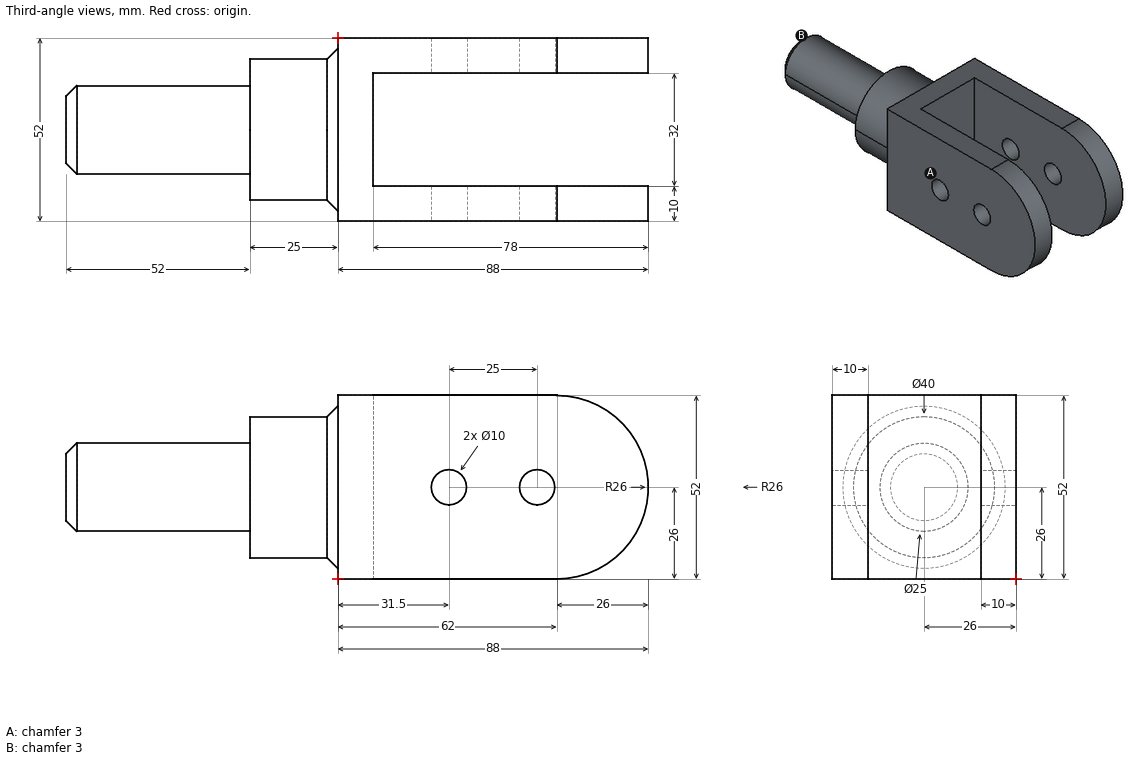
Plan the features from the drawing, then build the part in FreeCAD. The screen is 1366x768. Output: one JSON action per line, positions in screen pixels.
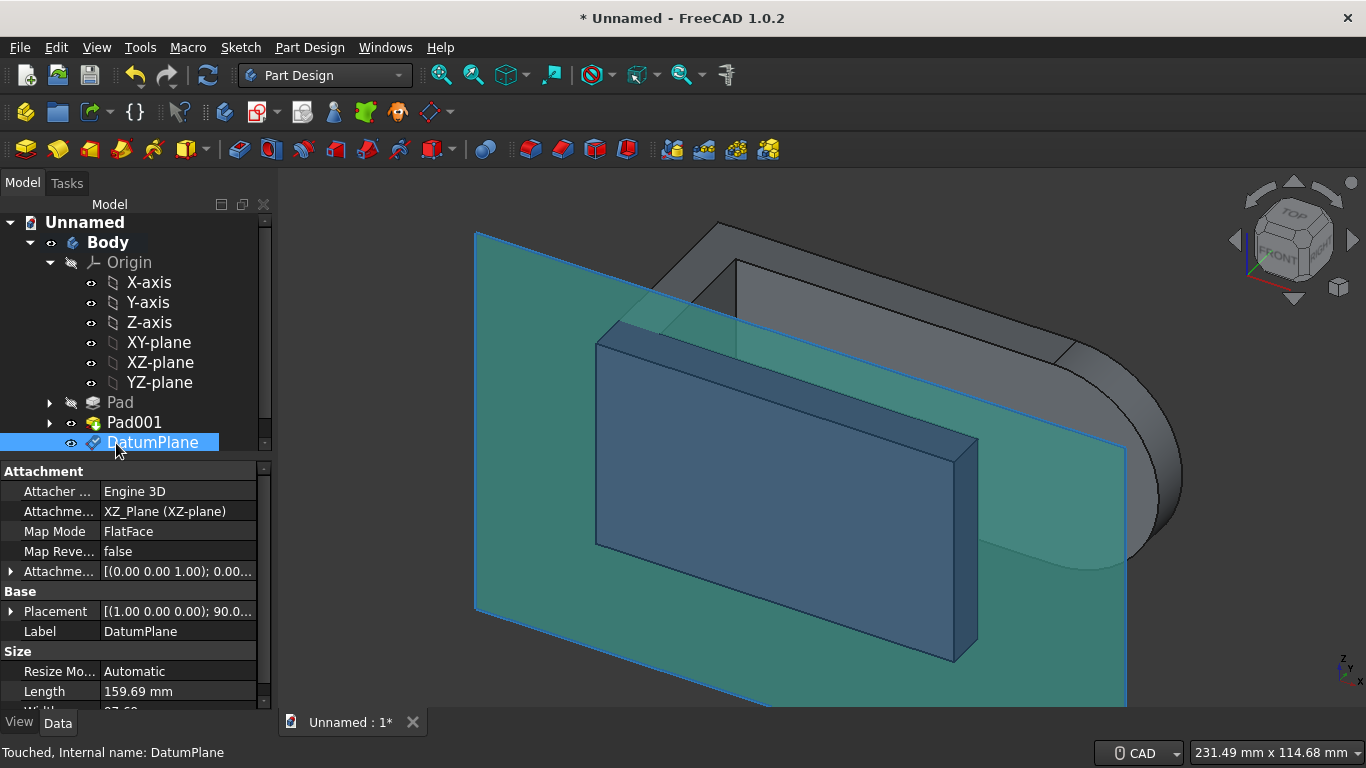
{"action": "left_click", "coordinate": [258, 112]}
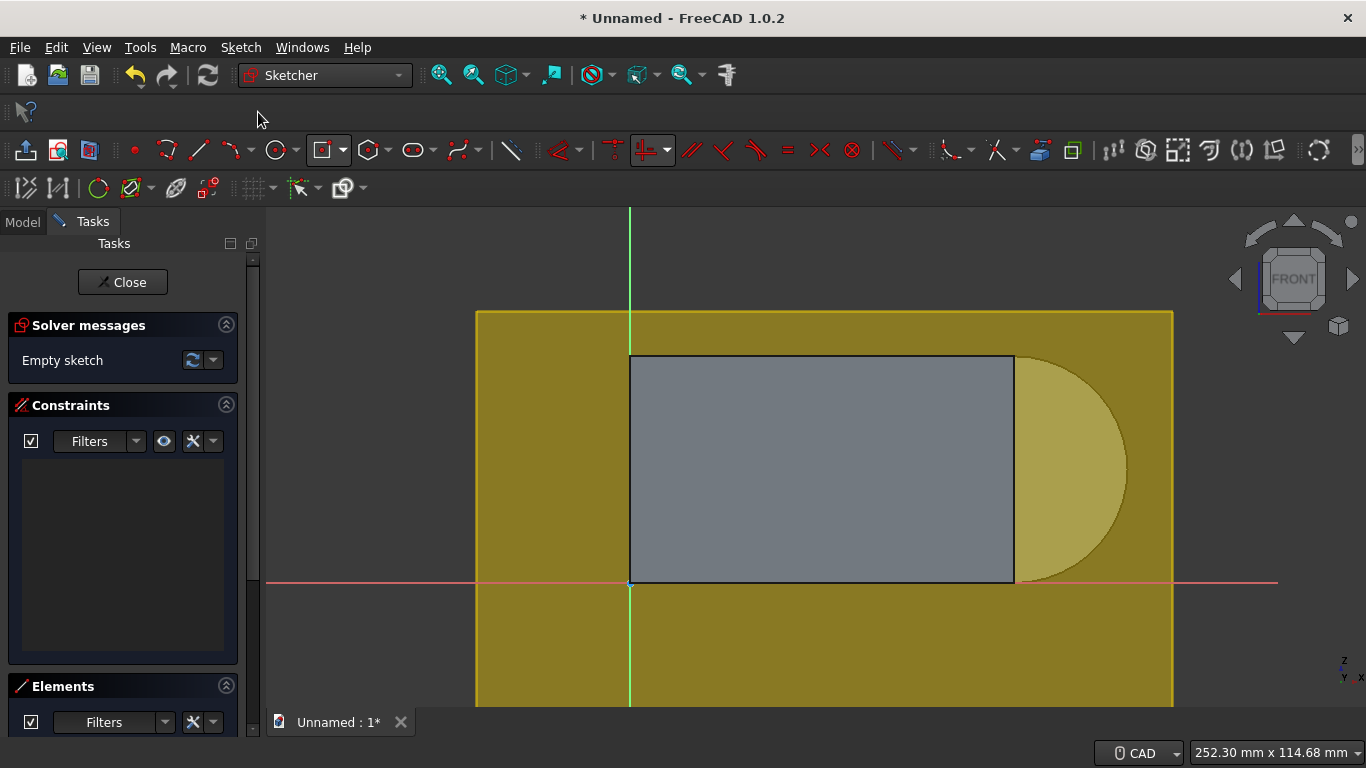
{"action": "left_click", "coordinate": [90, 150]}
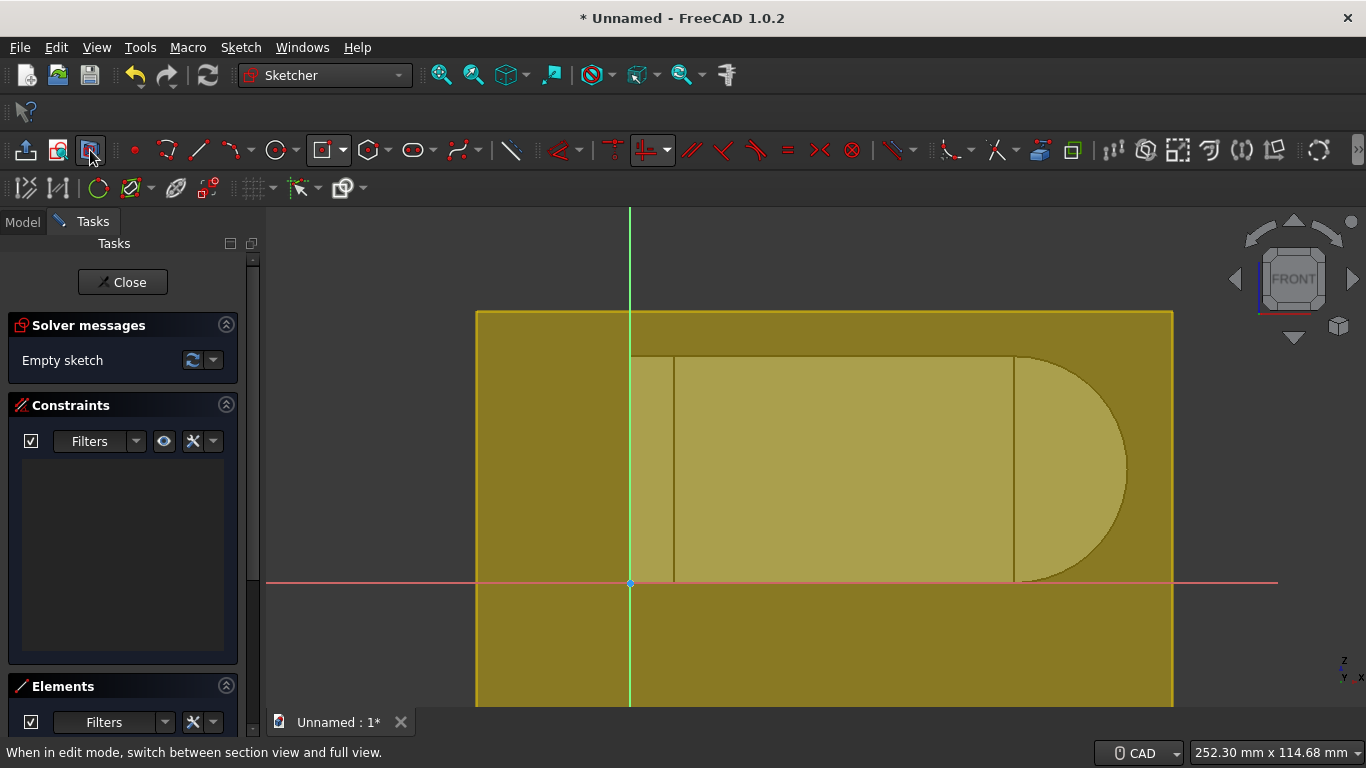
{"action": "left_click", "coordinate": [200, 150]}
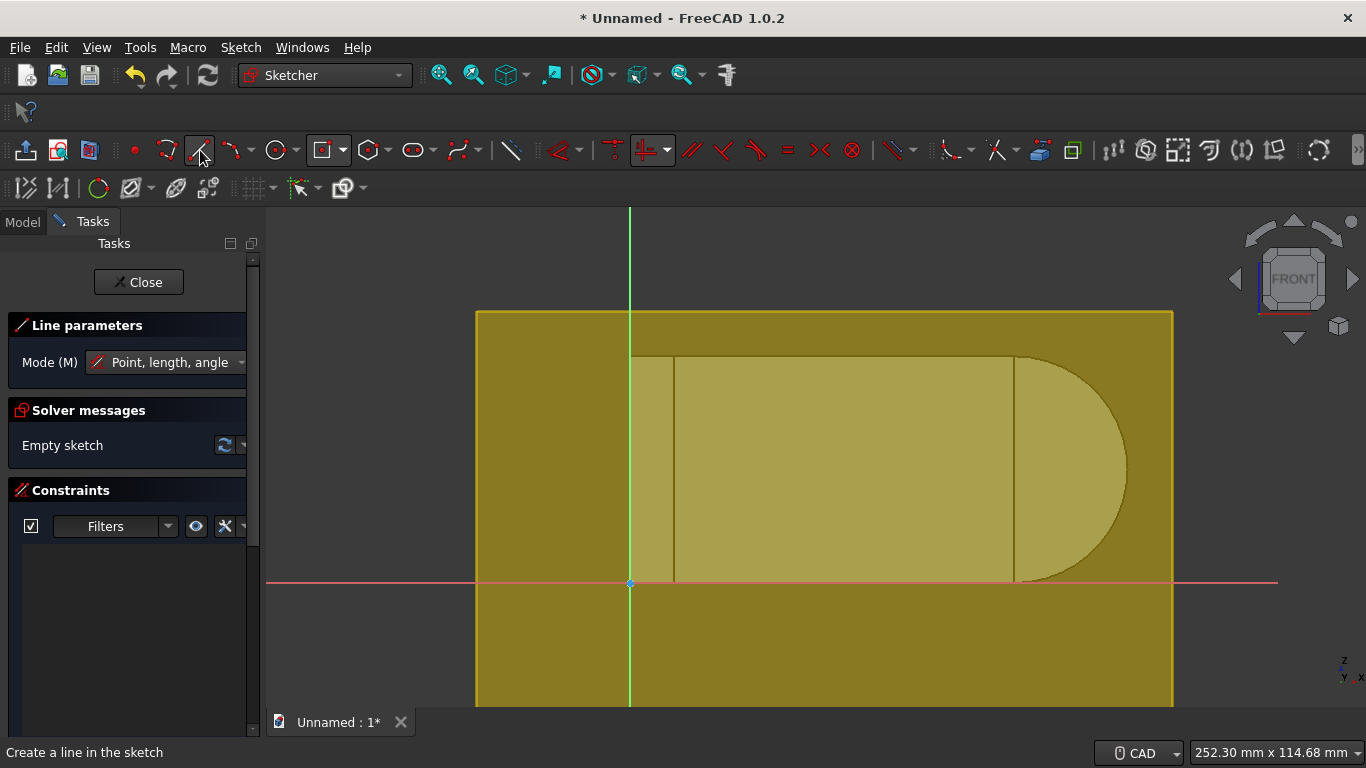
{"action": "left_click", "coordinate": [1014, 356]}
{"action": "left_click", "coordinate": [1014, 583]}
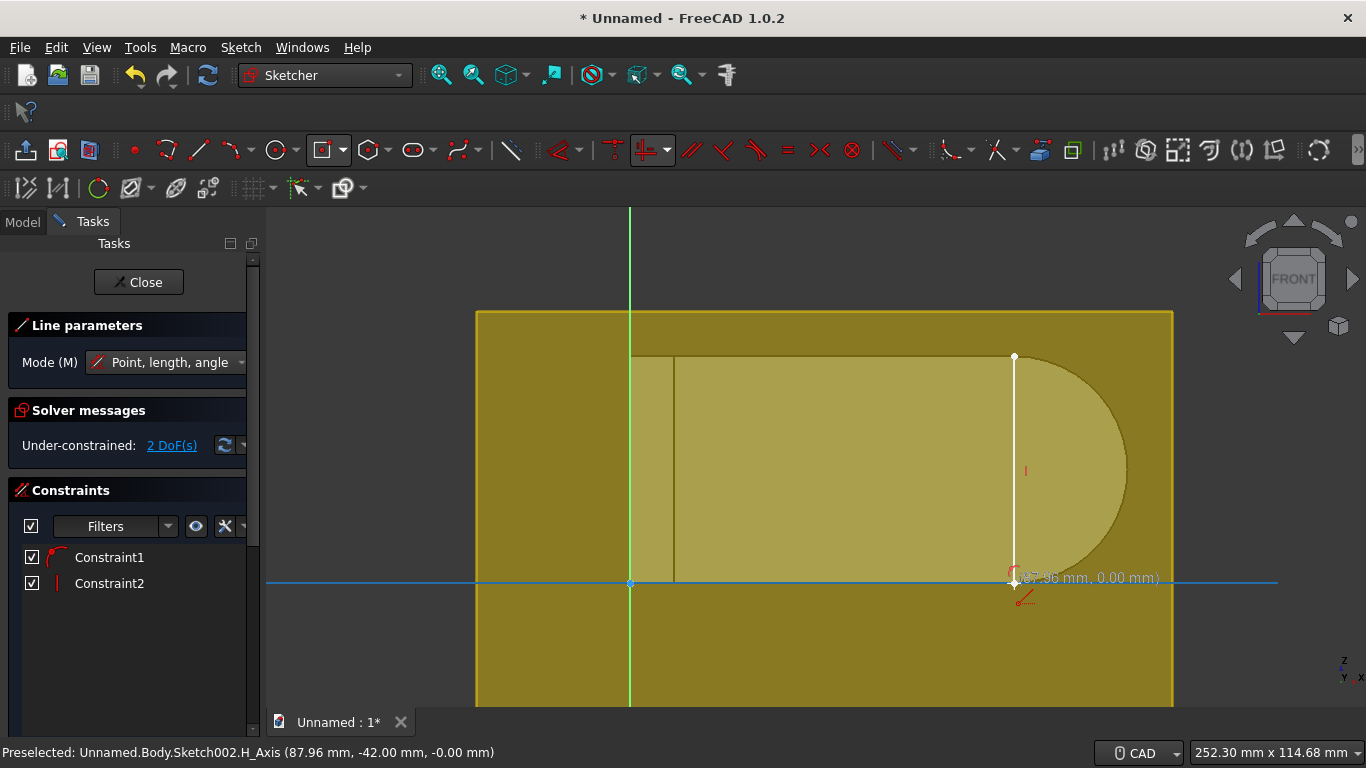
{"action": "left_click", "coordinate": [232, 150]}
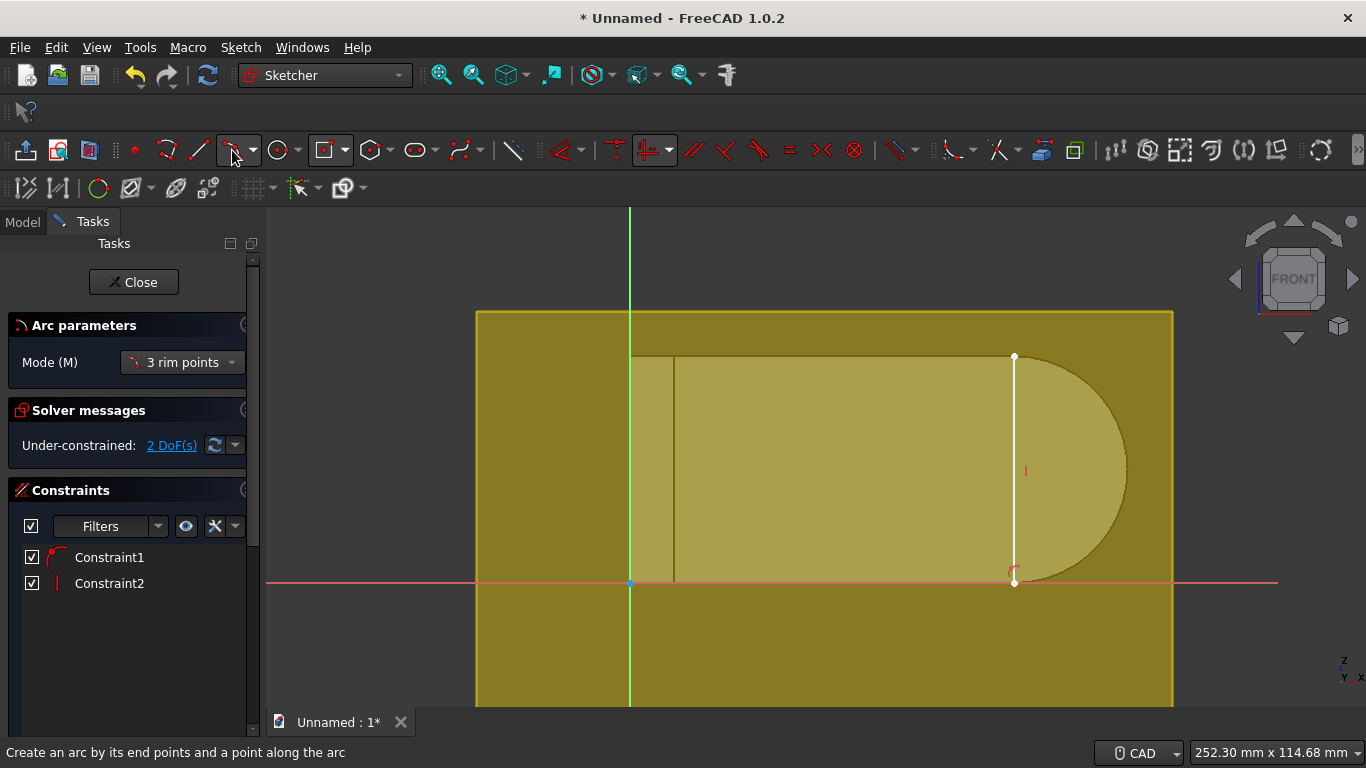
{"action": "left_click", "coordinate": [1014, 583]}
{"action": "left_click", "coordinate": [1014, 357]}
{"action": "left_click", "coordinate": [1128, 470]}
{"action": "key", "text": "Escape"}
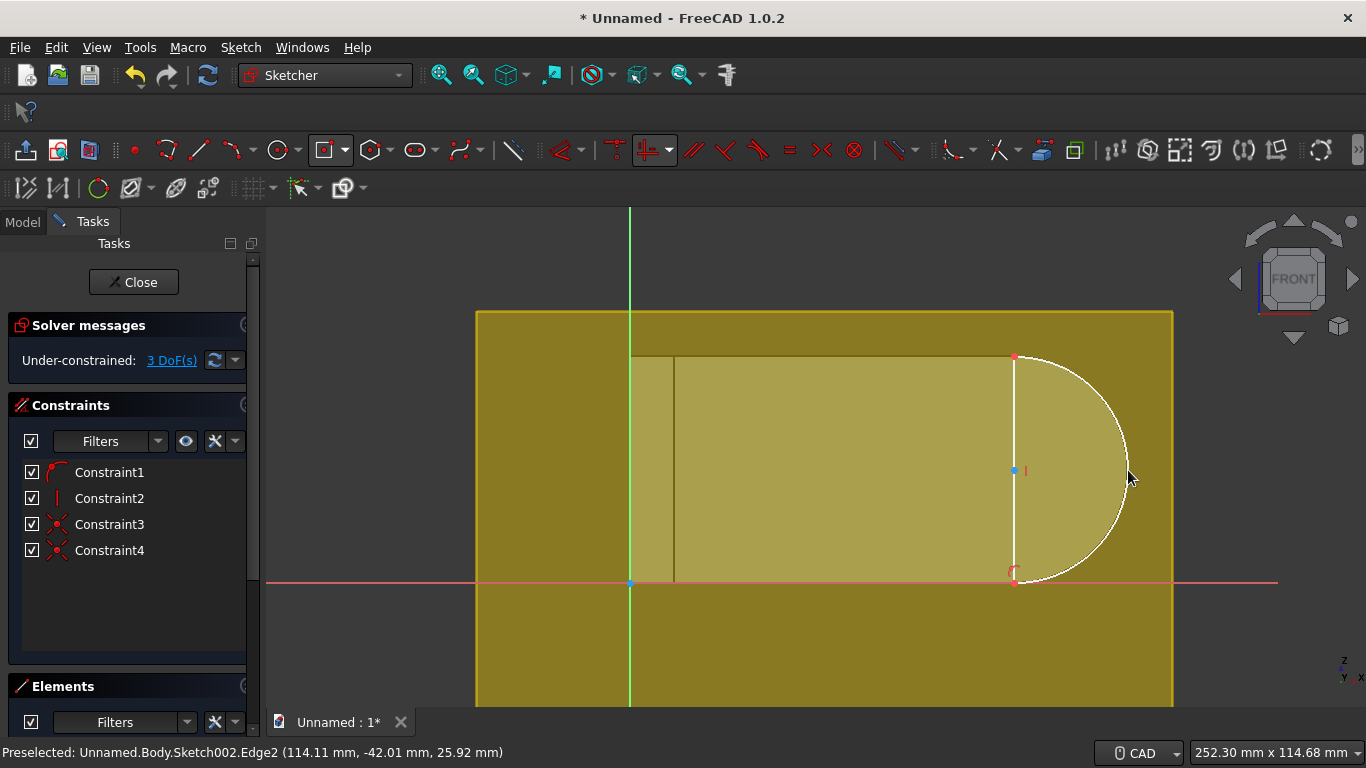
{"action": "left_click", "coordinate": [560, 150]}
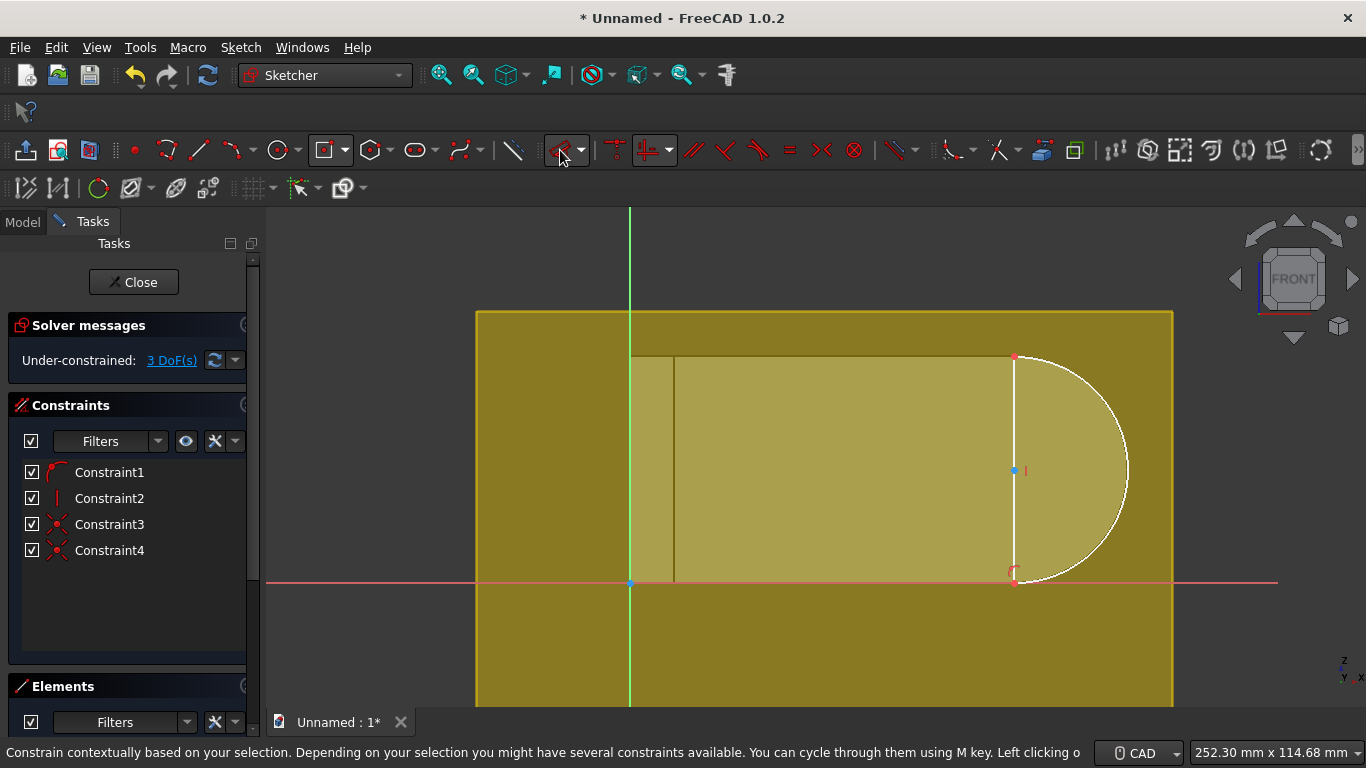
{"action": "left_click", "coordinate": [1106, 537]}
{"action": "left_click", "coordinate": [1132, 556]}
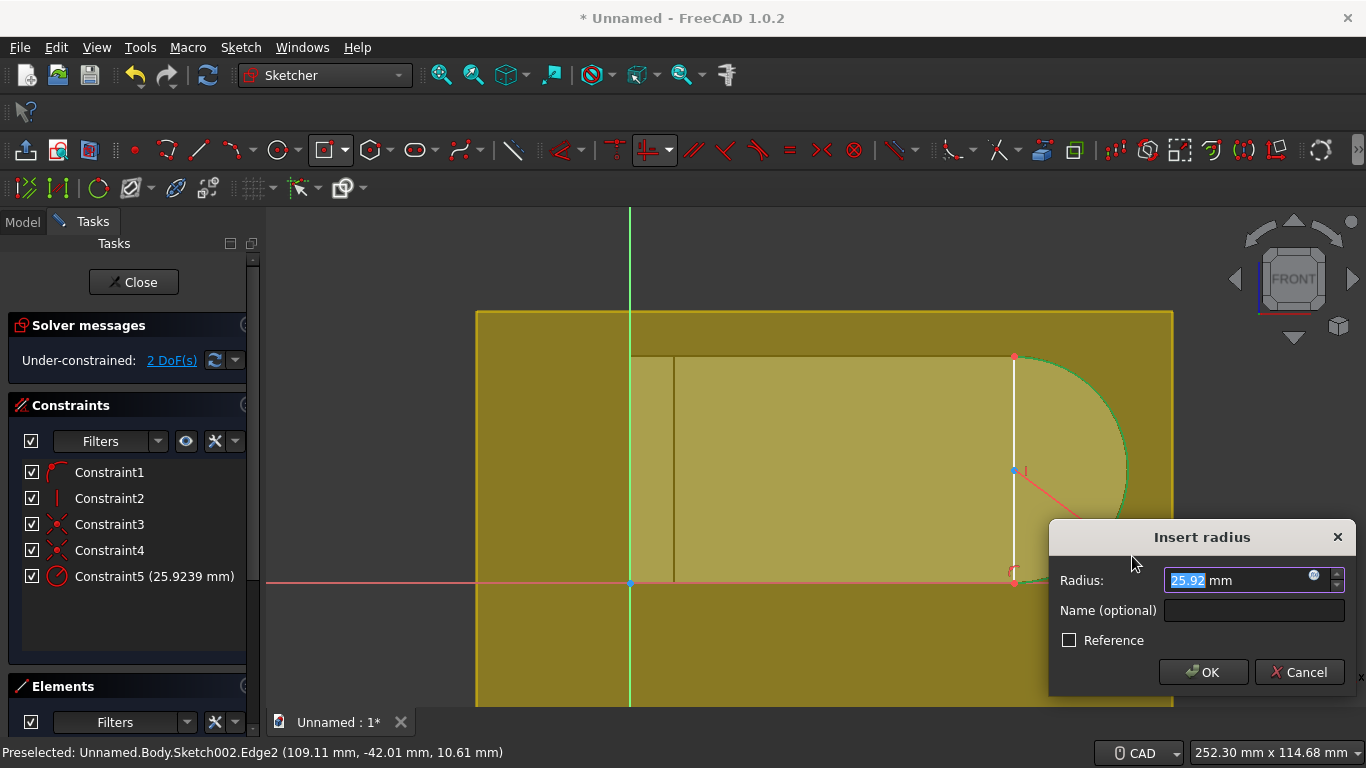
{"action": "type", "text": "26"}
{"action": "key", "text": "Return"}